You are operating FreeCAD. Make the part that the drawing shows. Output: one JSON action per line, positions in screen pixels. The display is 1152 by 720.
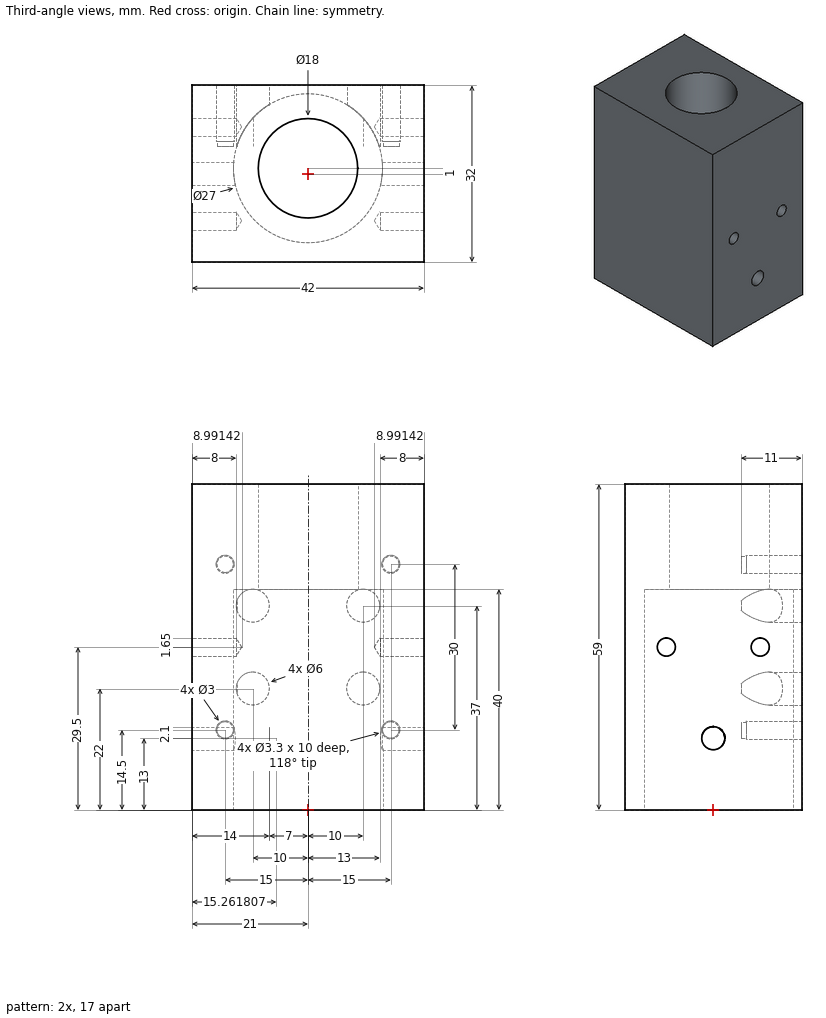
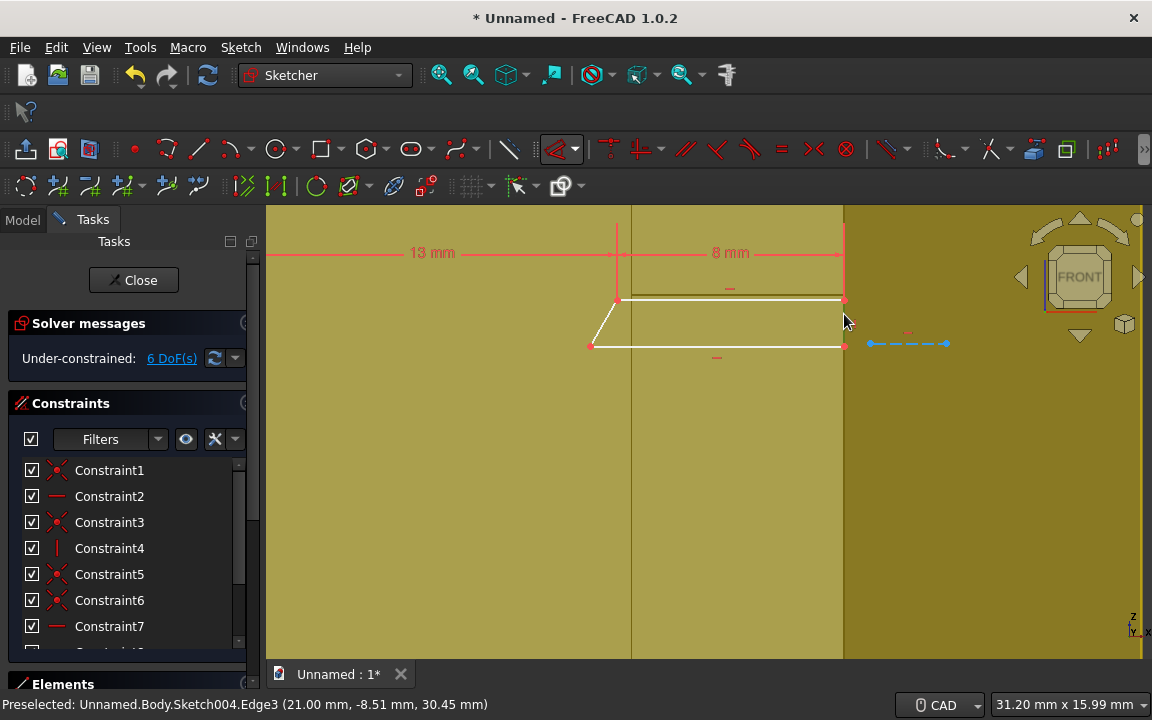
{"action": "key", "text": "i"}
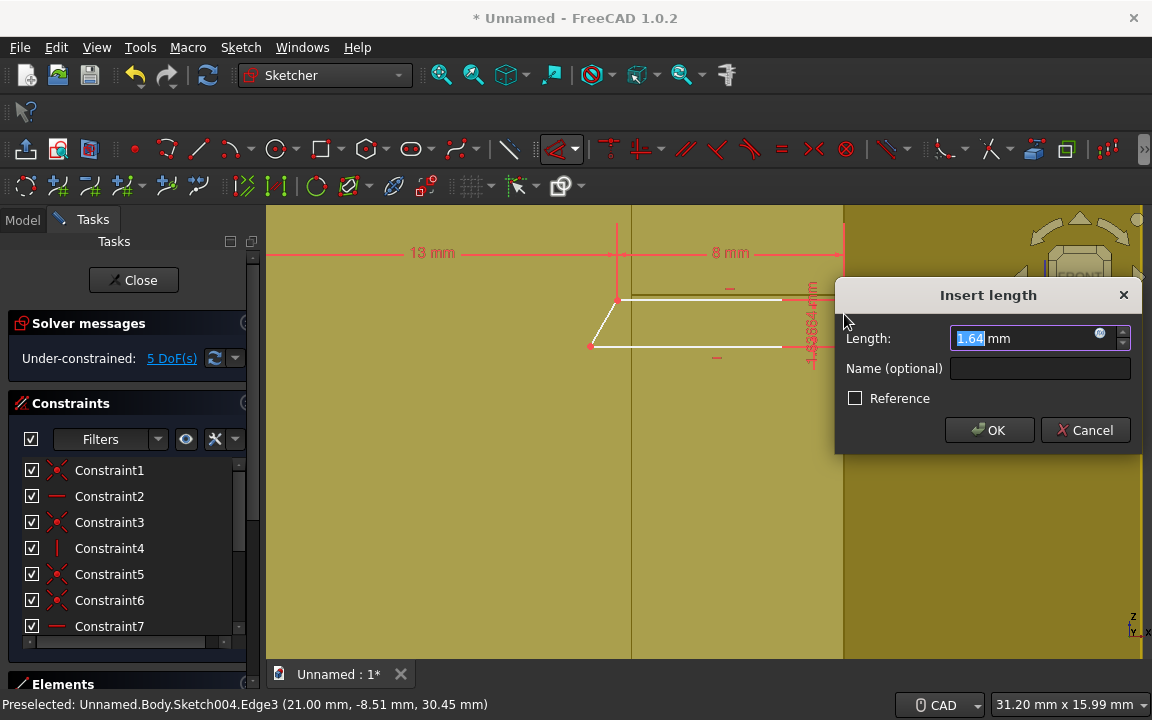
{"action": "type", "text": "1.65"}
{"action": "key", "text": "Return"}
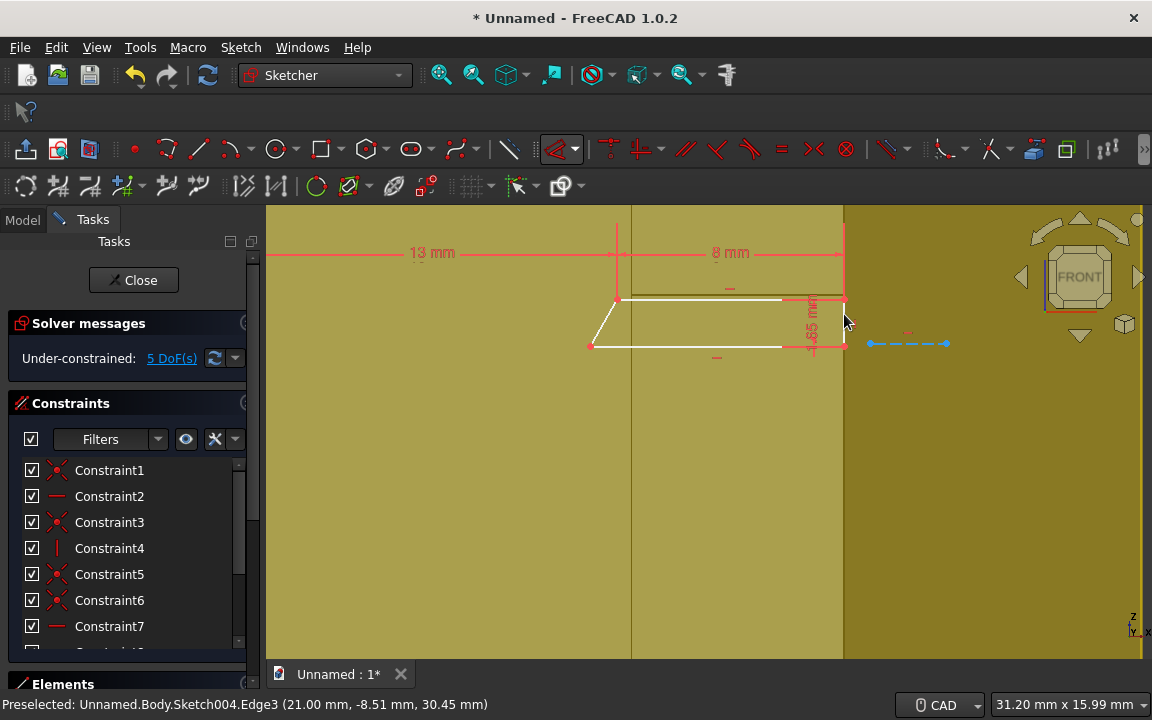
{"action": "left_click", "coordinate": [590, 347]}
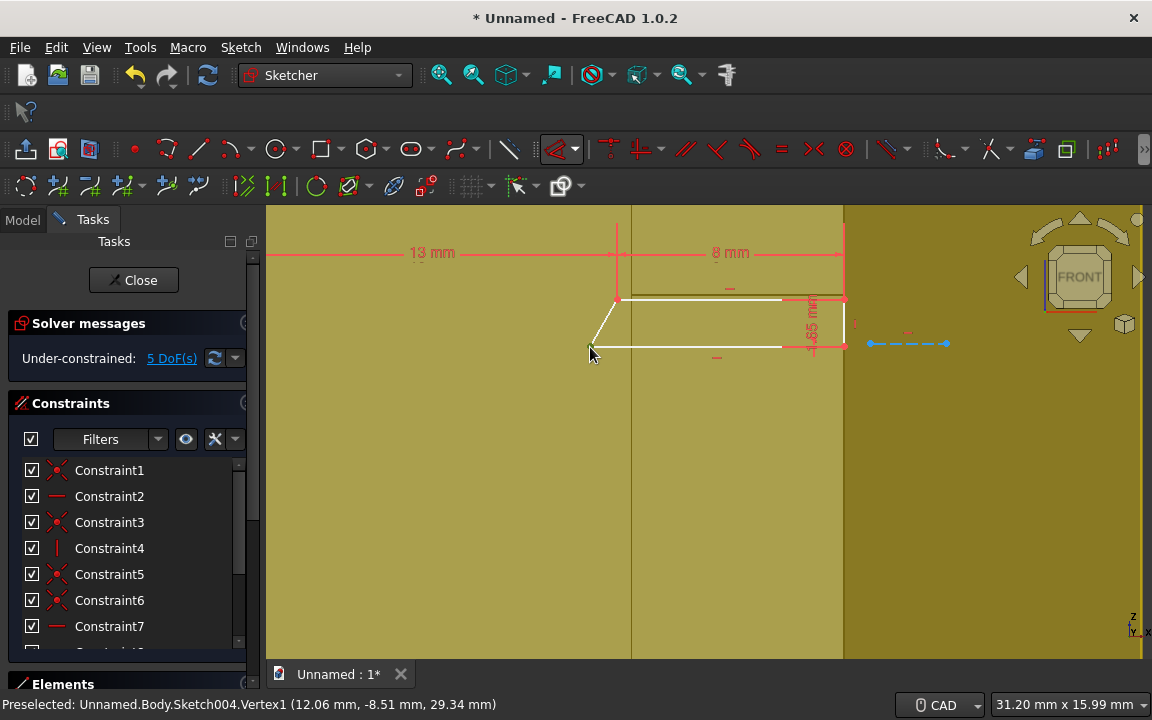
{"action": "left_click", "coordinate": [578, 150]}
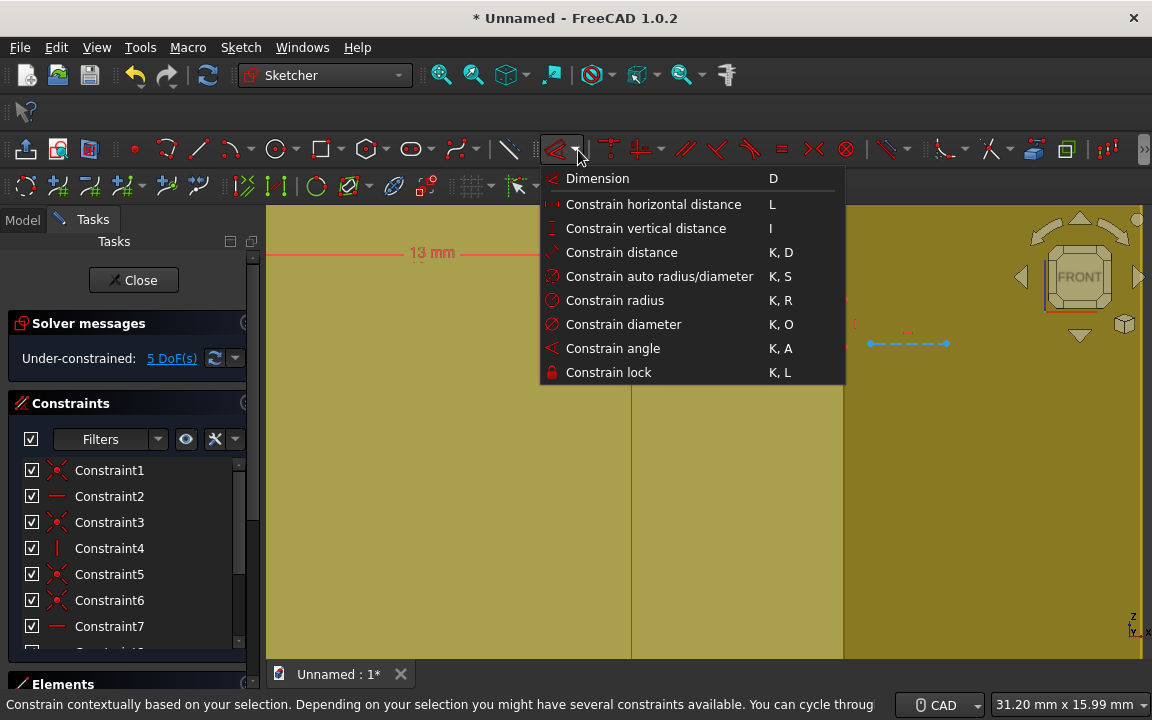
{"action": "left_click", "coordinate": [693, 228]}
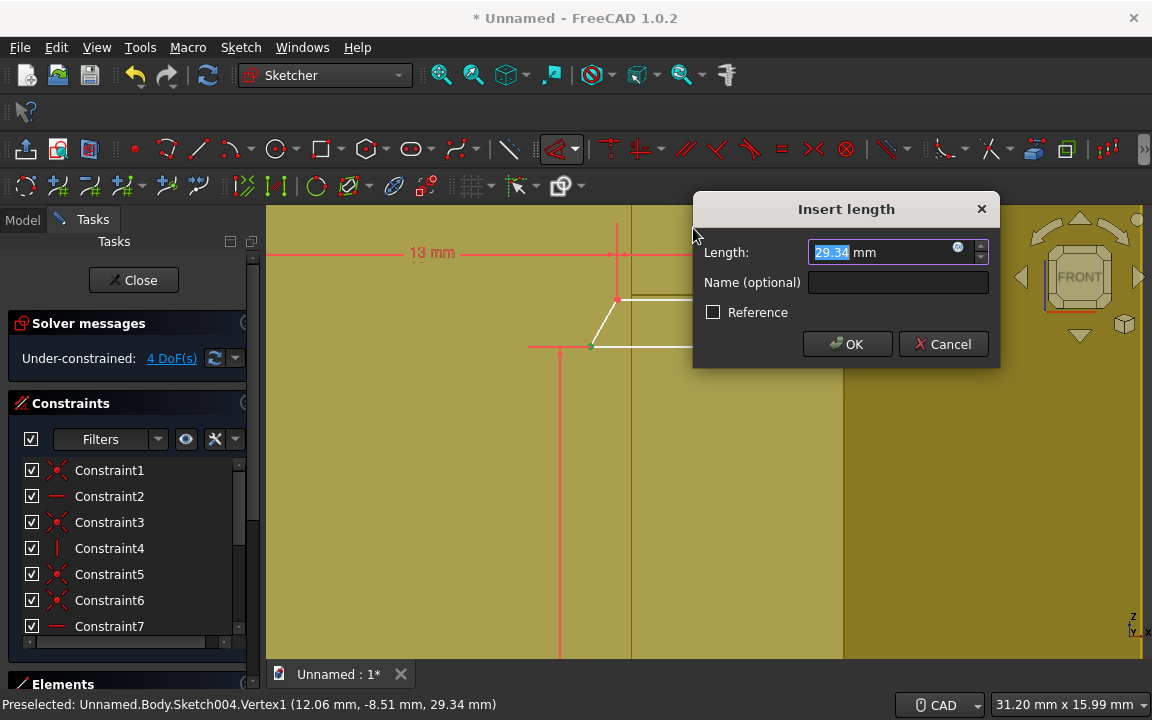
{"action": "type", "text": "29.5"}
{"action": "key", "text": "Return"}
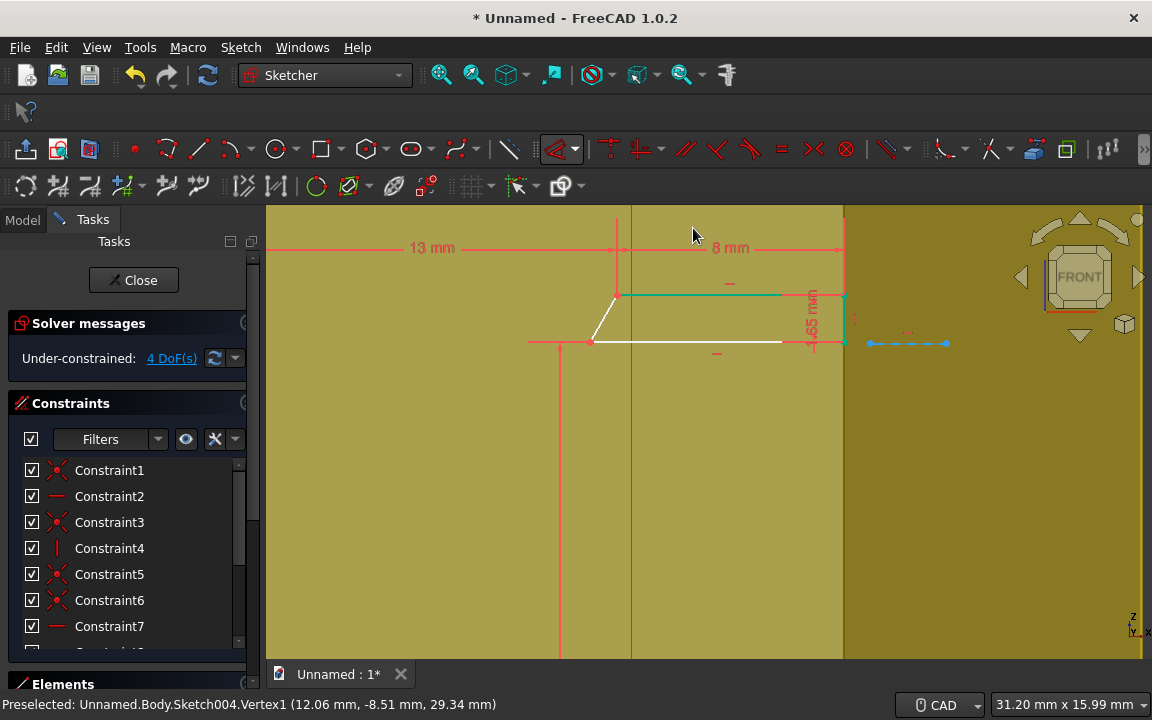
{"action": "left_click", "coordinate": [870, 344]}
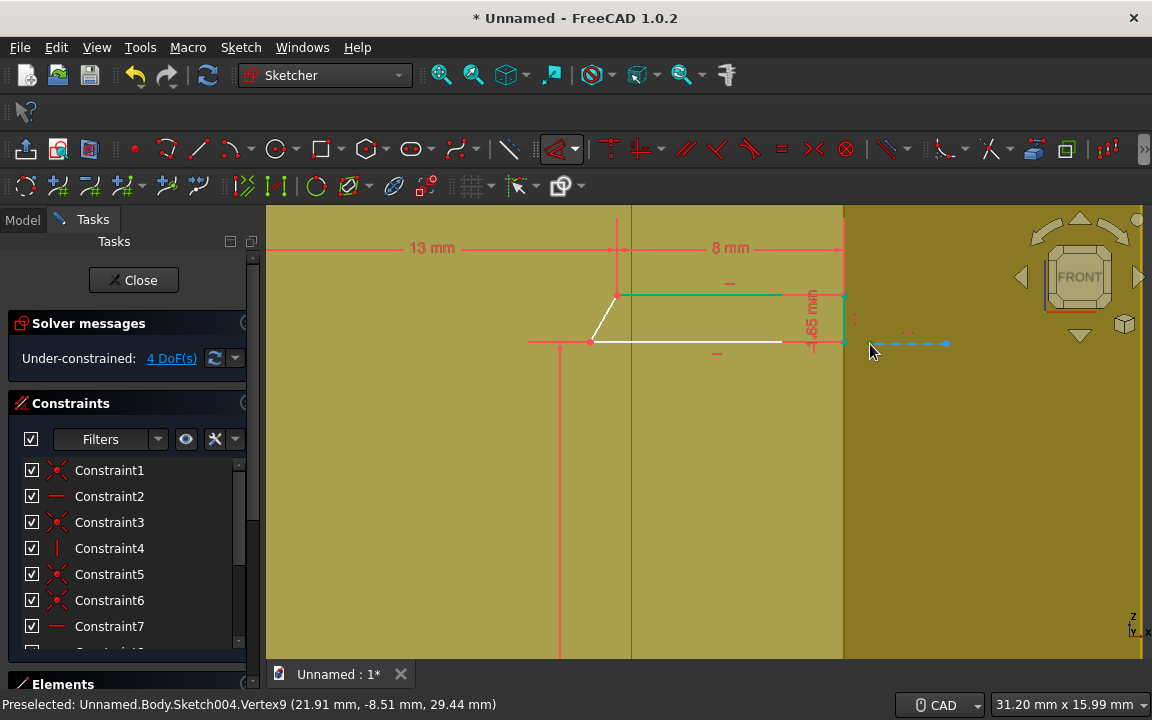
{"action": "key", "text": "i"}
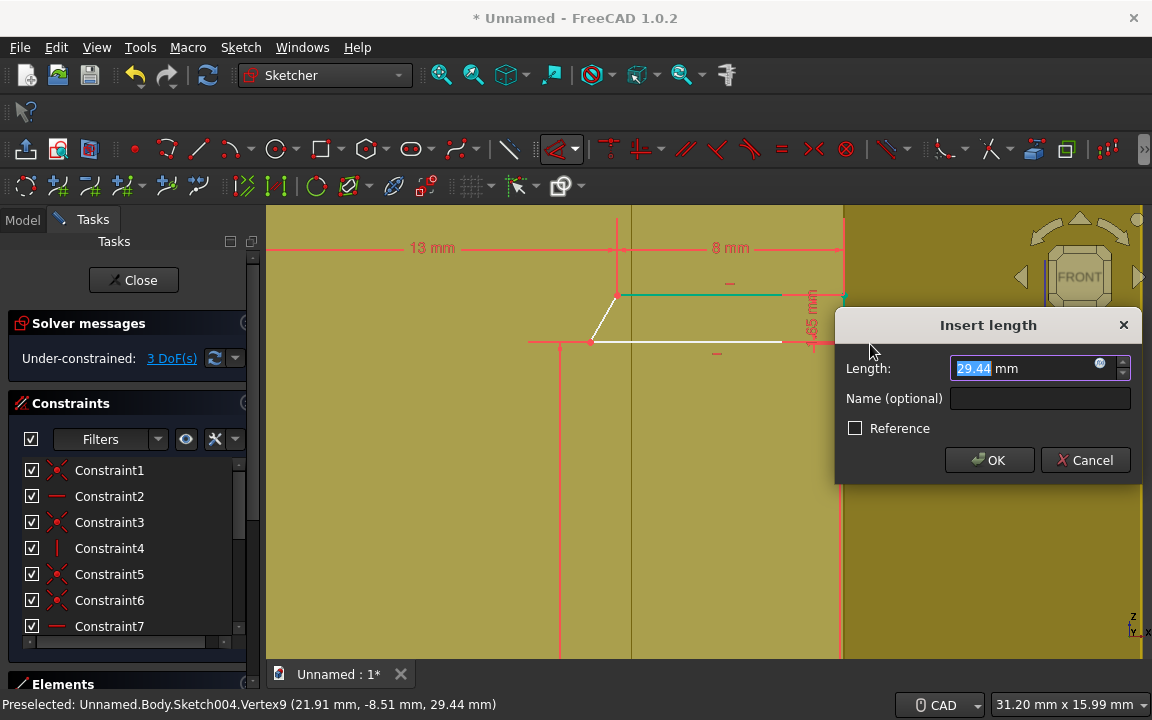
{"action": "type", "text": "29.5"}
{"action": "key", "text": "Return"}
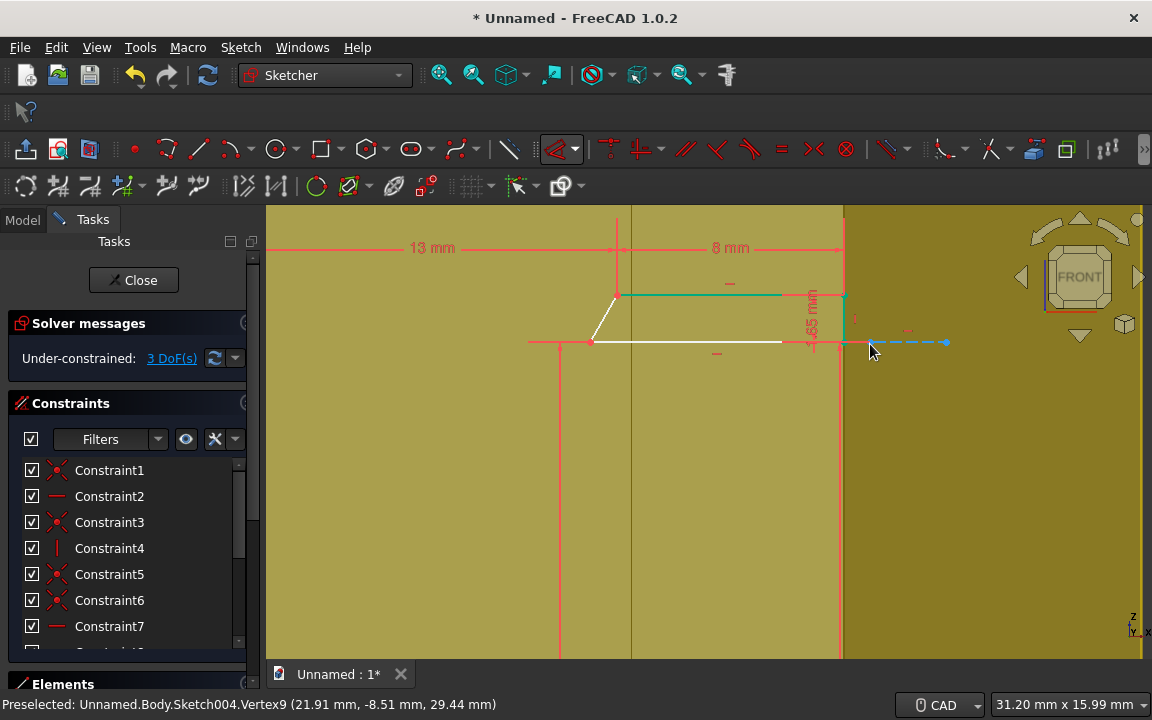
{"action": "left_click", "coordinate": [768, 342]}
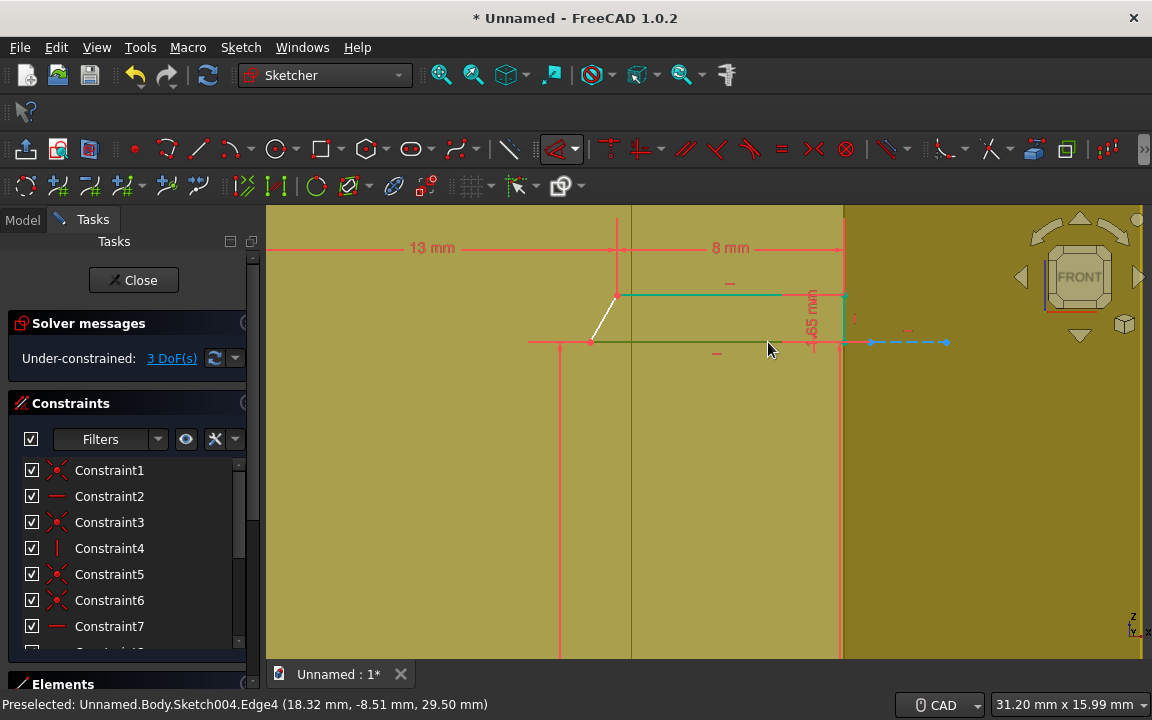
{"action": "key", "text": "l"}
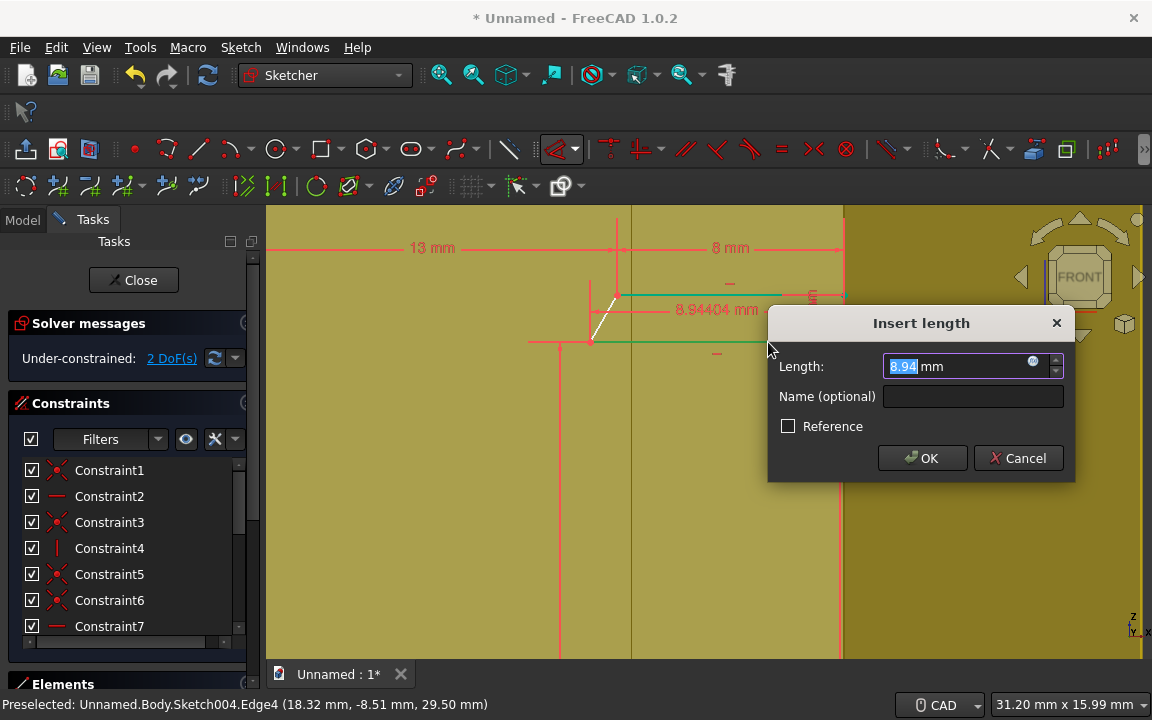
{"action": "type", "text": "8.99142"}
{"action": "key", "text": "Return"}